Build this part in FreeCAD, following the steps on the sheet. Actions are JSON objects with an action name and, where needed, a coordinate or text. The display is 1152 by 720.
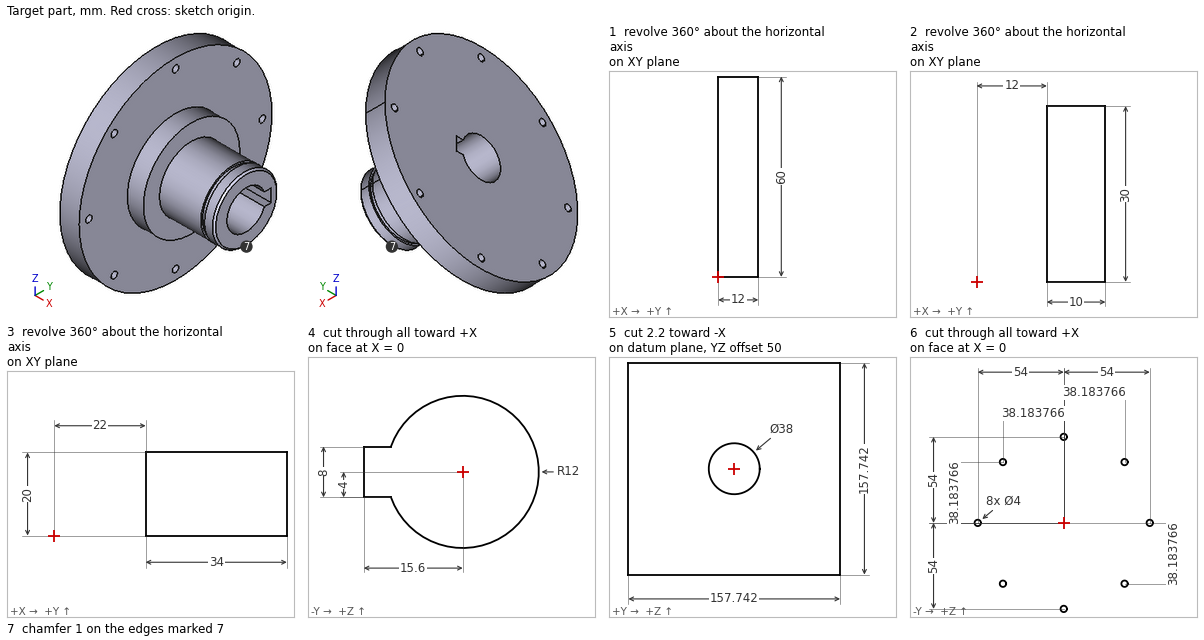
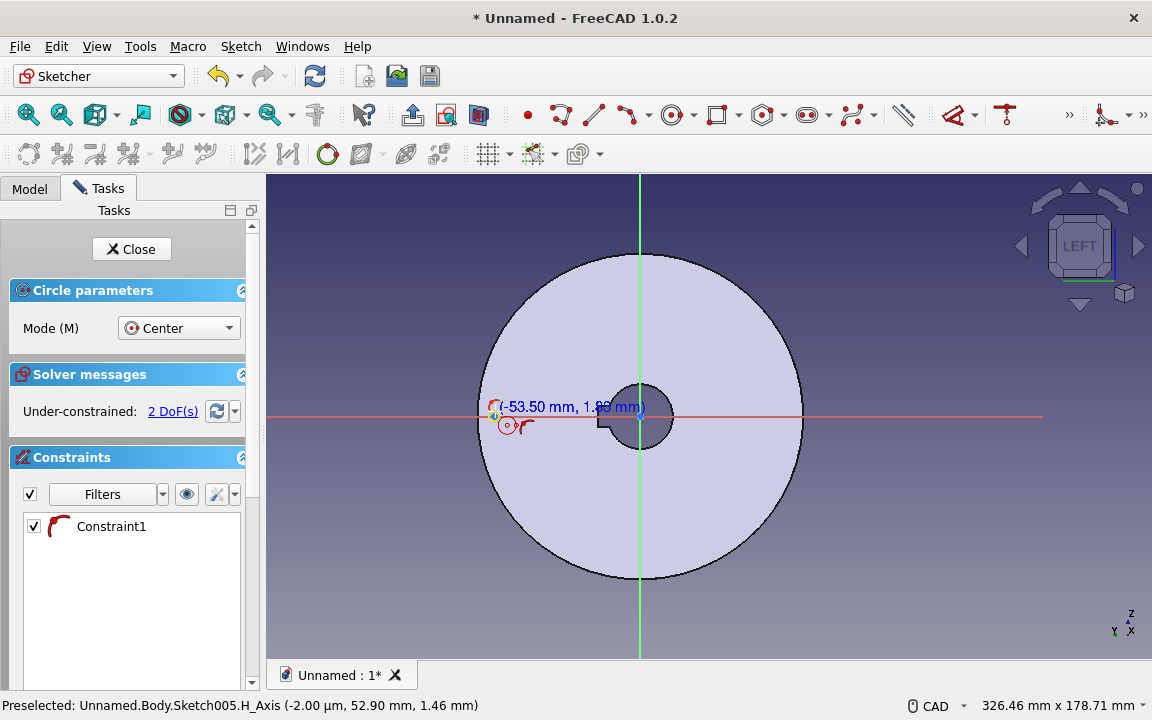
{"action": "scroll", "coordinate": [537, 313], "scroll_direction": "up", "scroll_amount": 8}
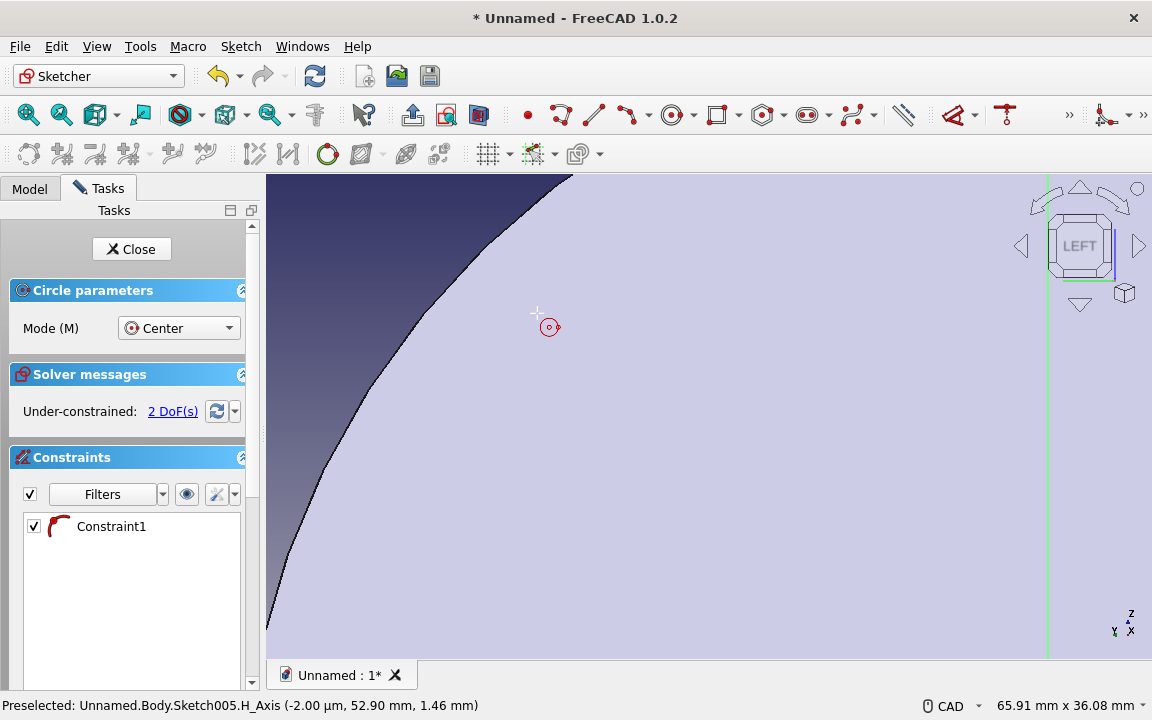
{"action": "scroll", "coordinate": [537, 313], "scroll_direction": "down", "scroll_amount": 8}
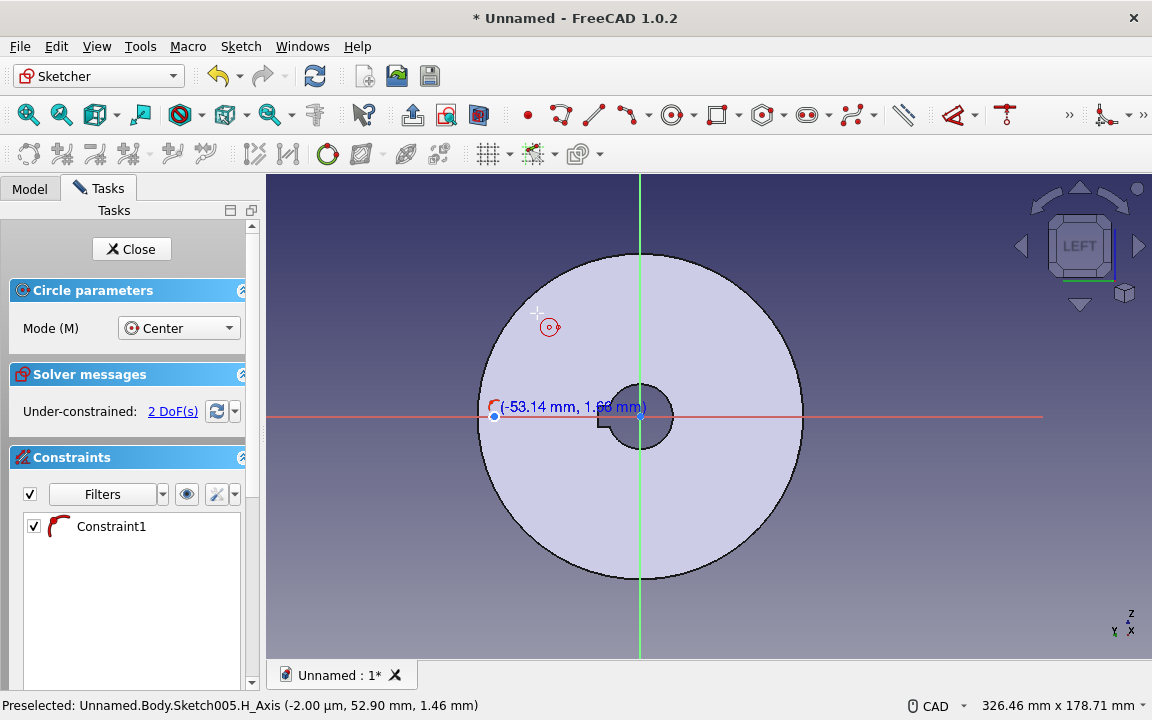
{"action": "left_click", "coordinate": [537, 313]}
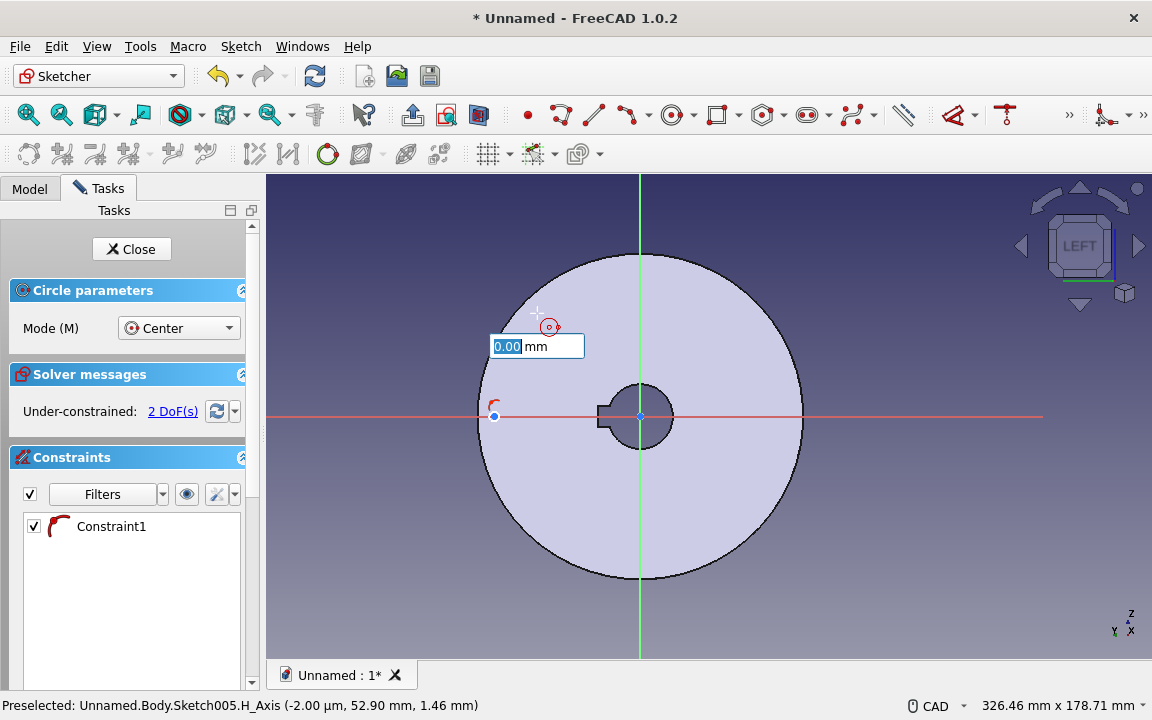
{"action": "scroll", "coordinate": [541, 309], "scroll_direction": "up", "scroll_amount": 6}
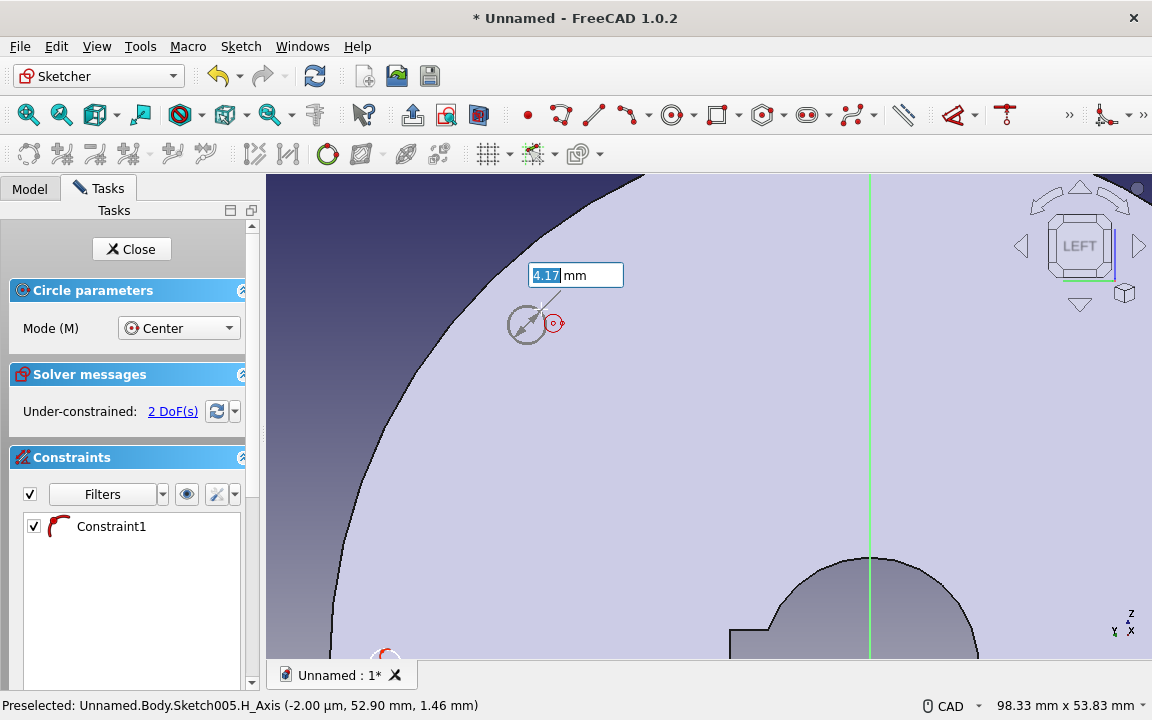
{"action": "left_click", "coordinate": [539, 309]}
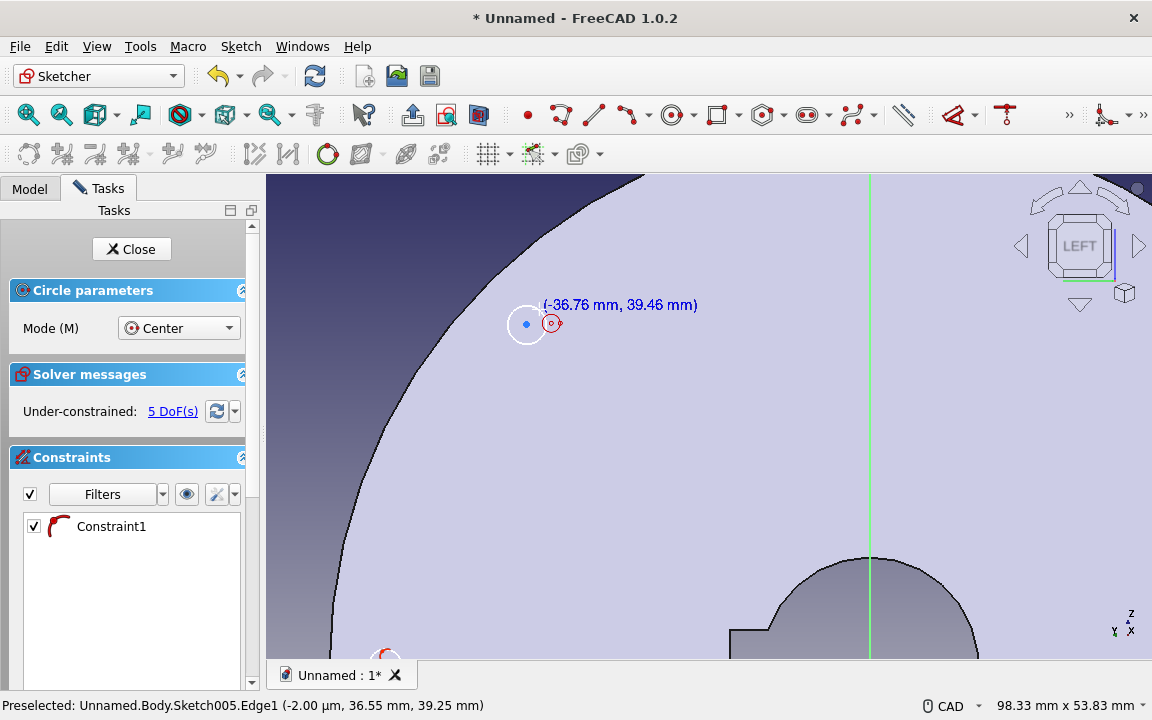
{"action": "scroll", "coordinate": [541, 309], "scroll_direction": "down", "scroll_amount": 6}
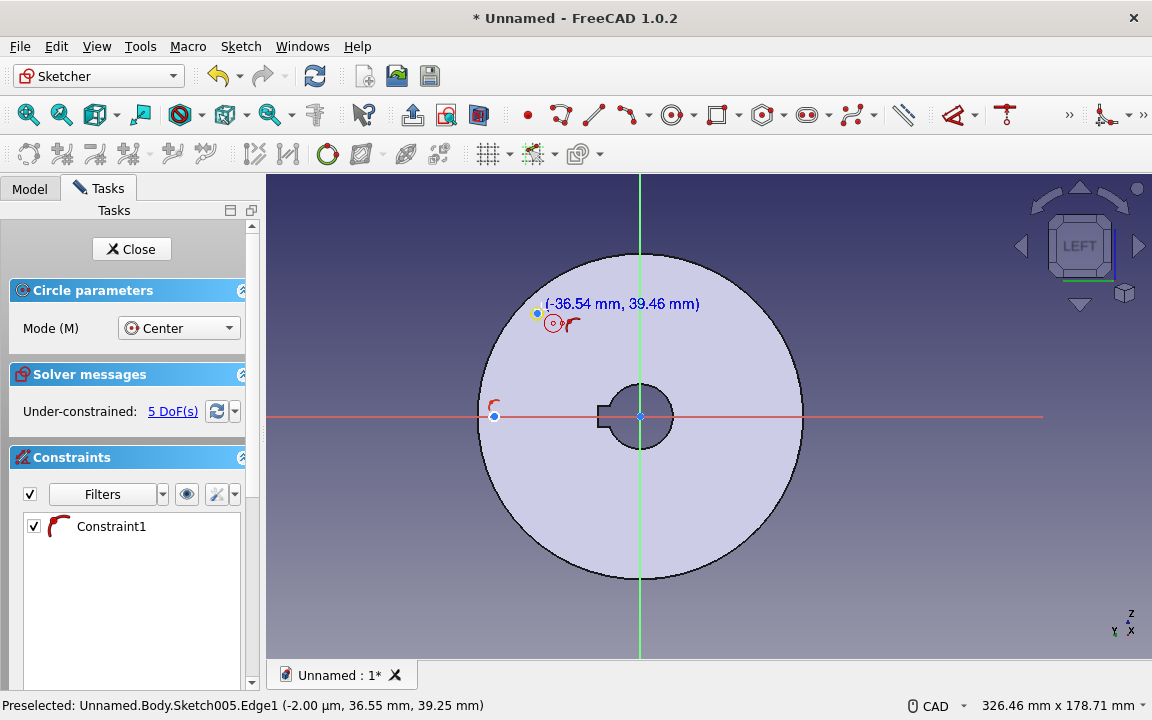
{"action": "scroll", "coordinate": [640, 270], "scroll_direction": "up", "scroll_amount": 8}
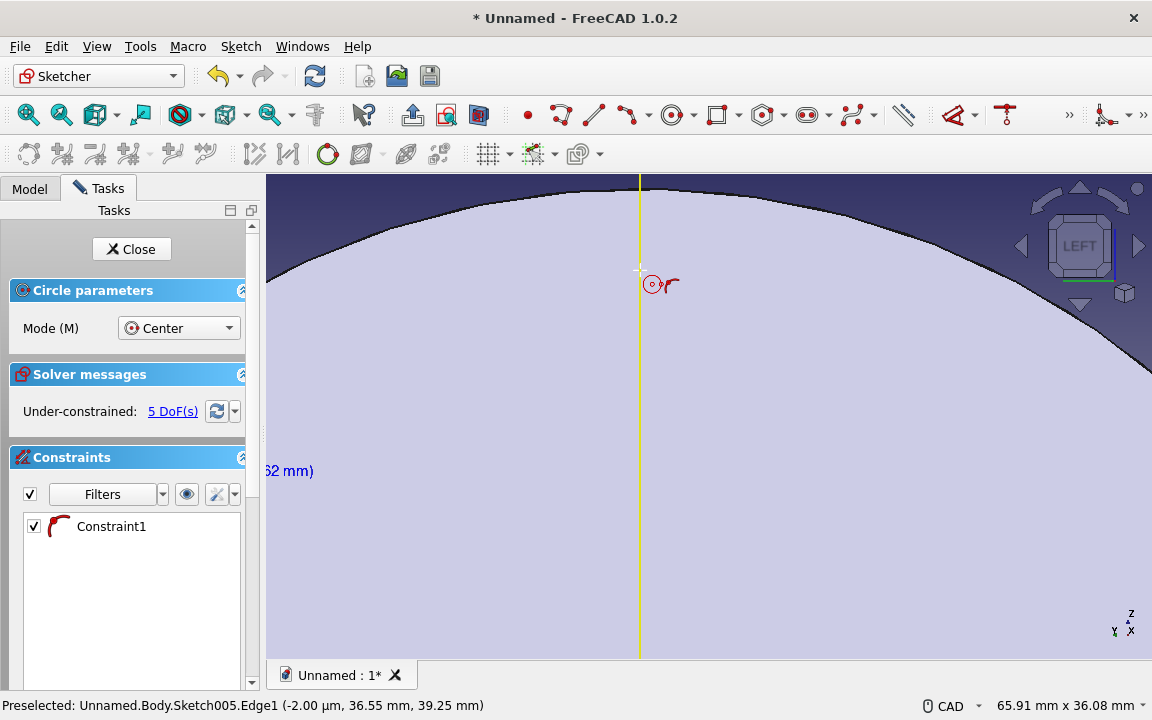
{"action": "scroll", "coordinate": [641, 270], "scroll_direction": "down", "scroll_amount": 8}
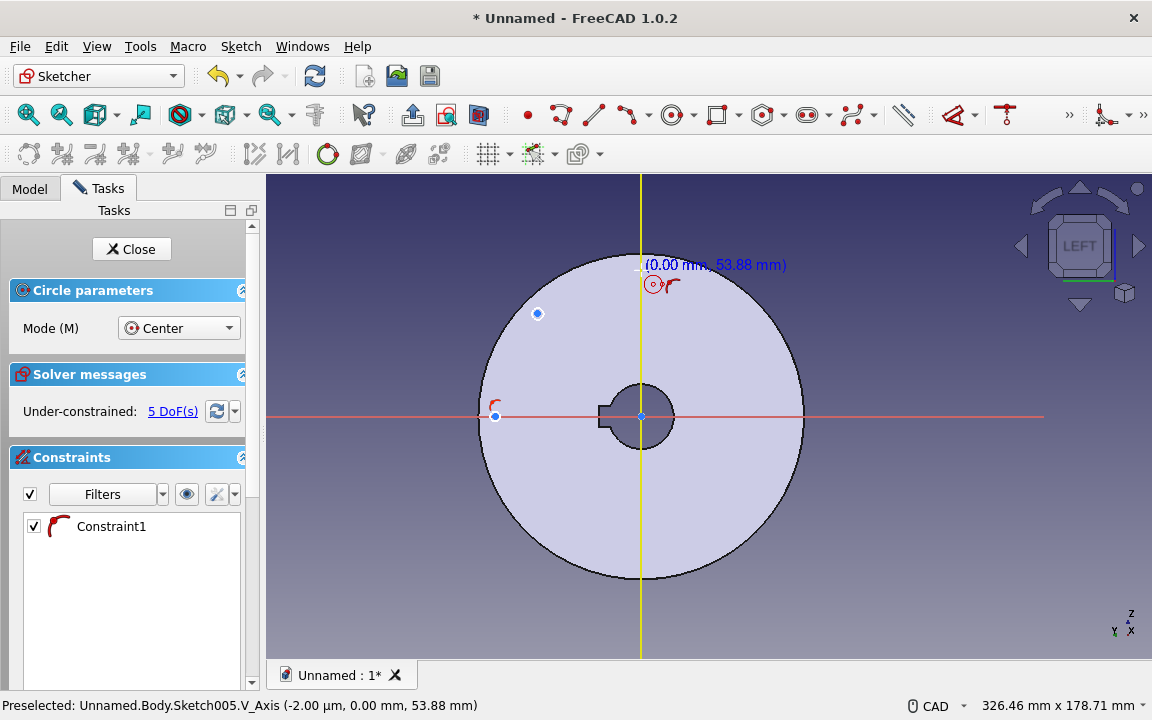
{"action": "left_click", "coordinate": [641, 270]}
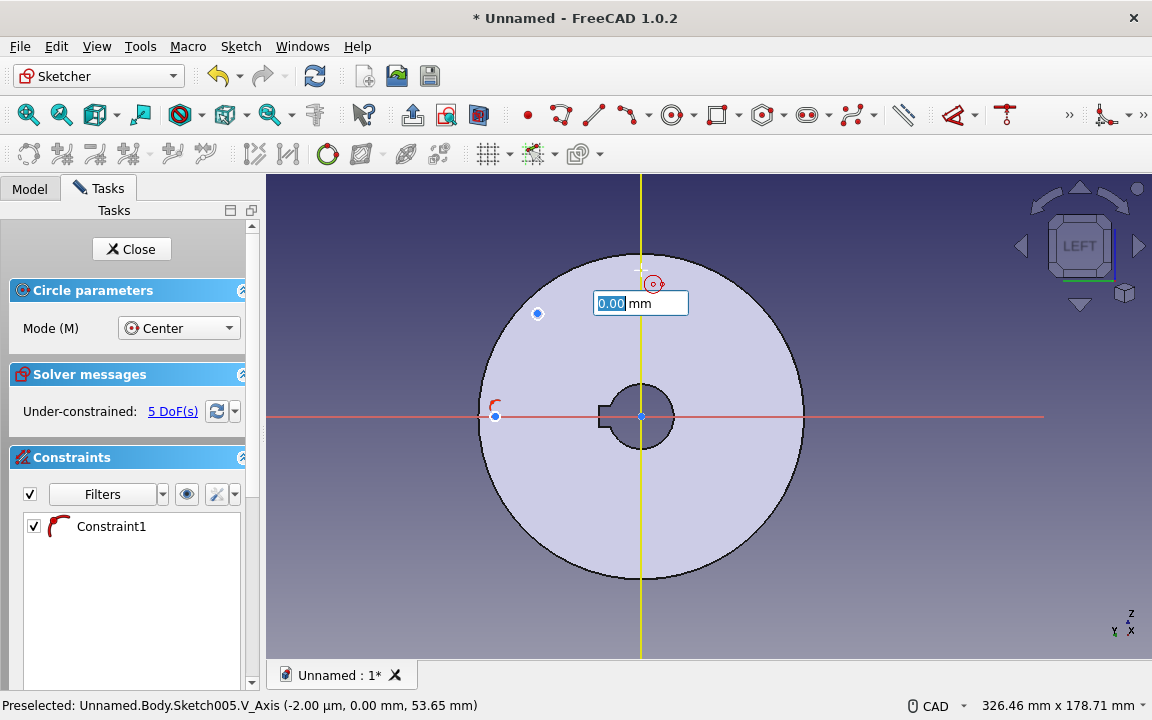
{"action": "scroll", "coordinate": [646, 268], "scroll_direction": "up", "scroll_amount": 6}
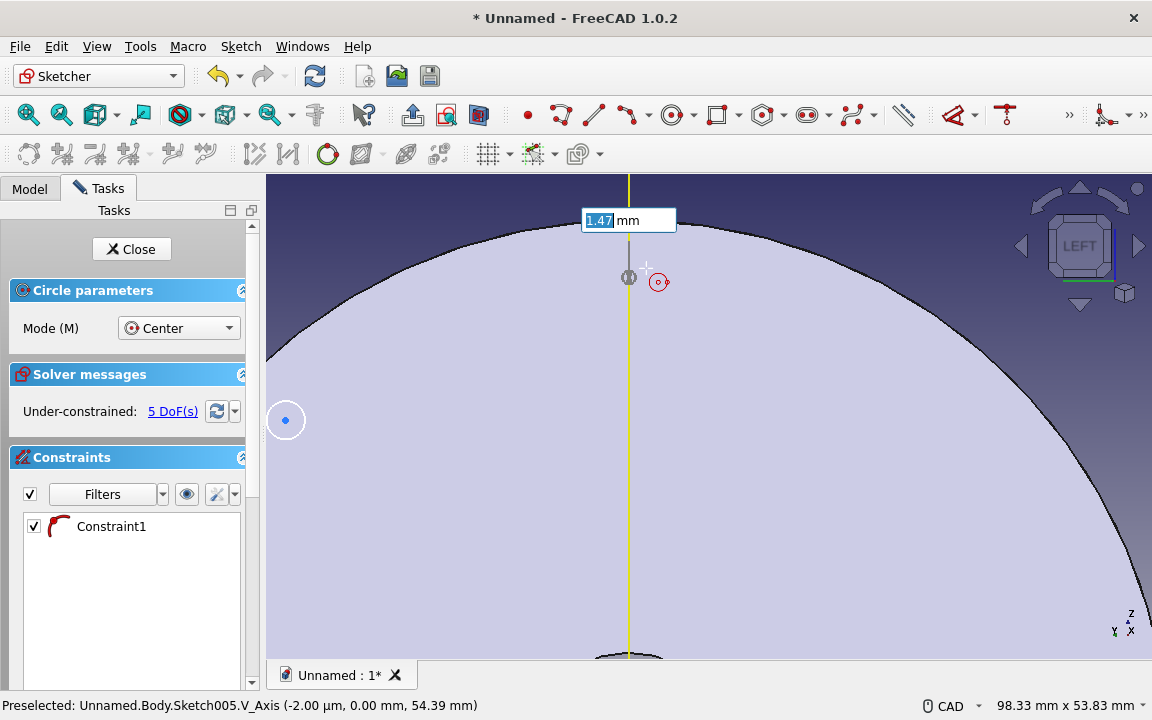
{"action": "left_click", "coordinate": [646, 268]}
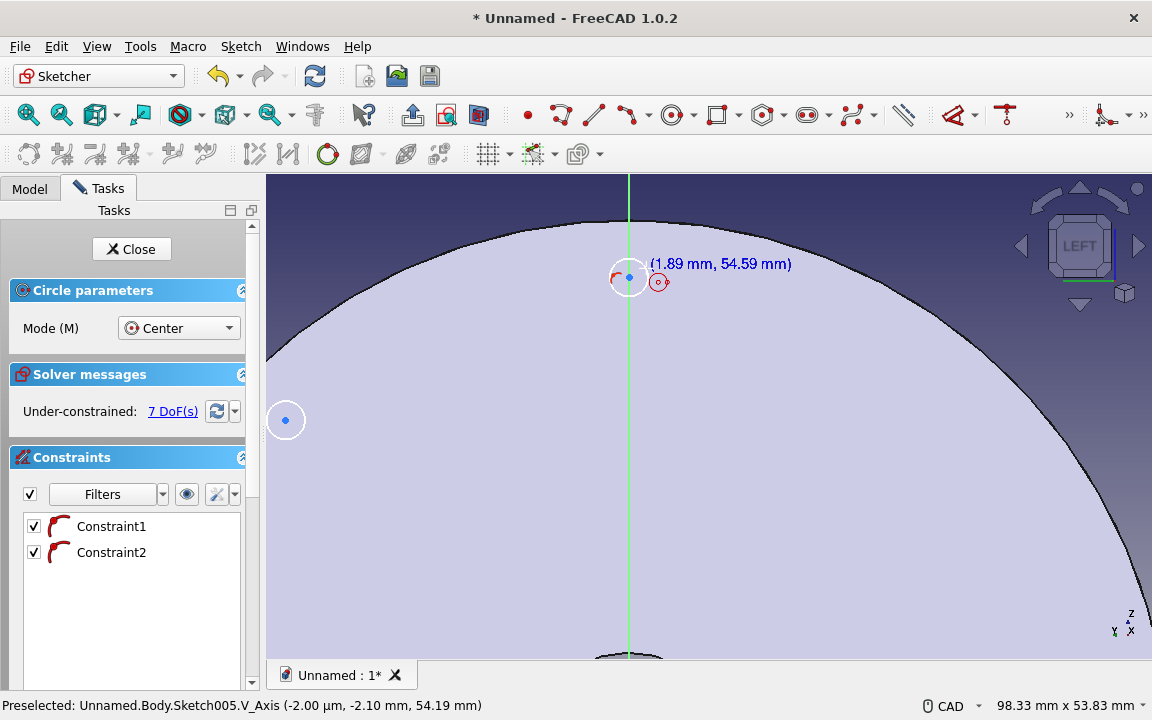
{"action": "scroll", "coordinate": [973, 417], "scroll_direction": "up", "scroll_amount": 2}